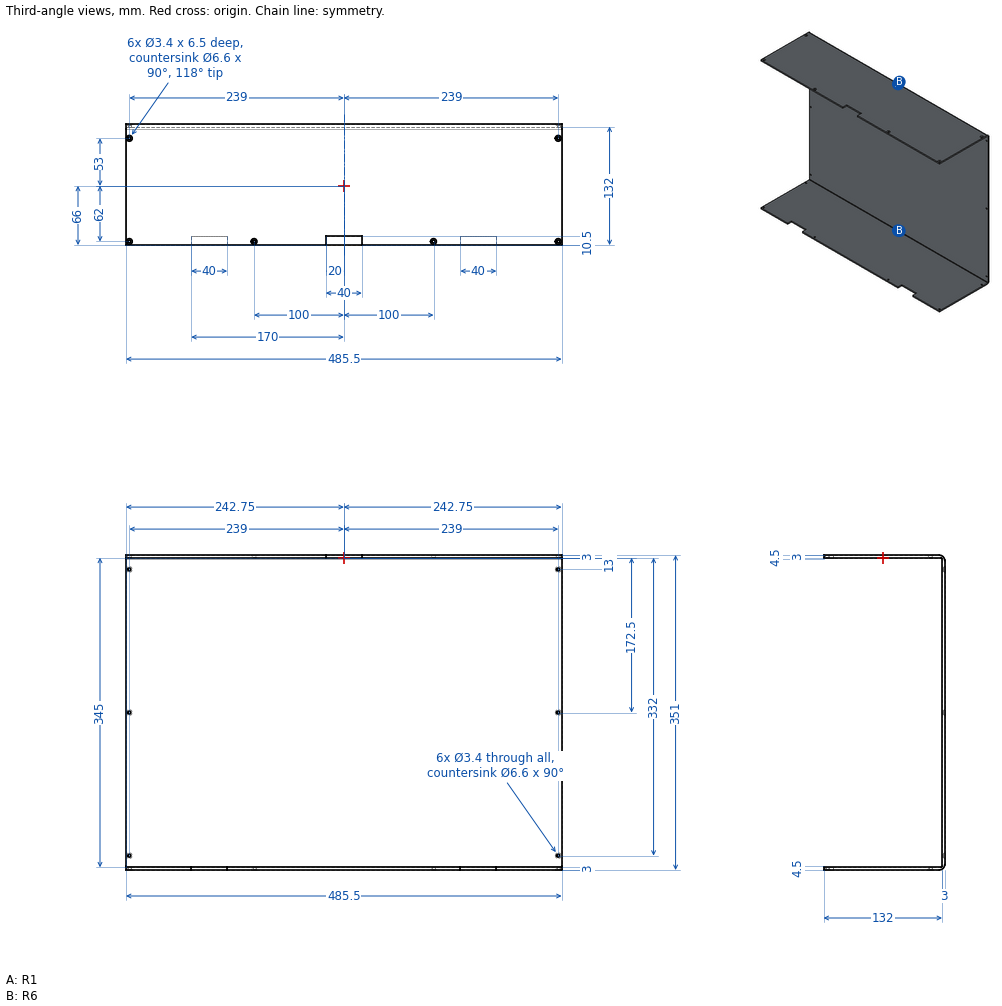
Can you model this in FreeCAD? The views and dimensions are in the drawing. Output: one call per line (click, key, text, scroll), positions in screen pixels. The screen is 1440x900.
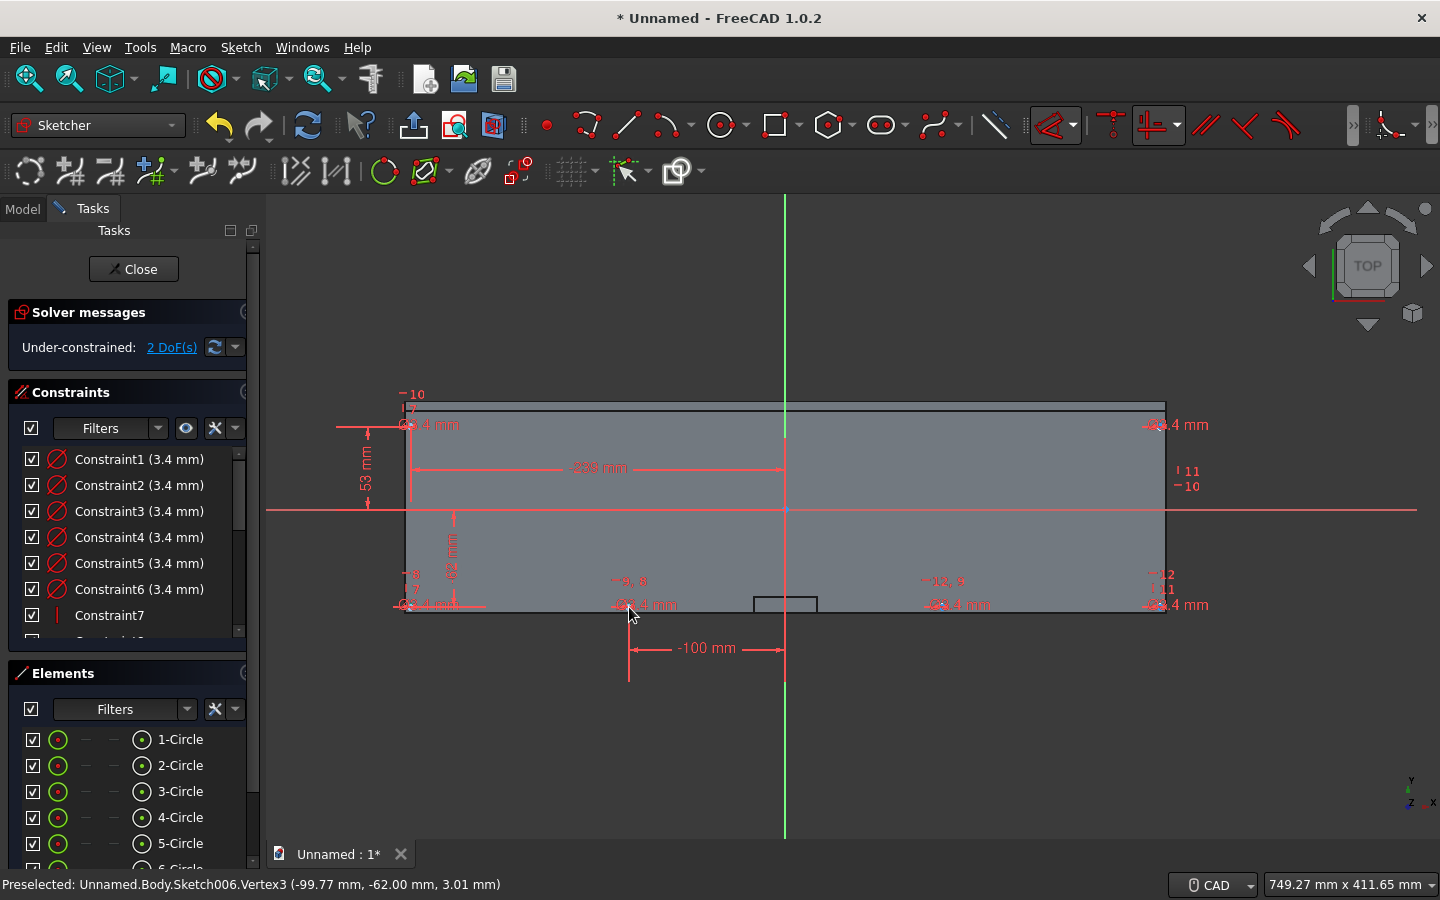
click(942, 607)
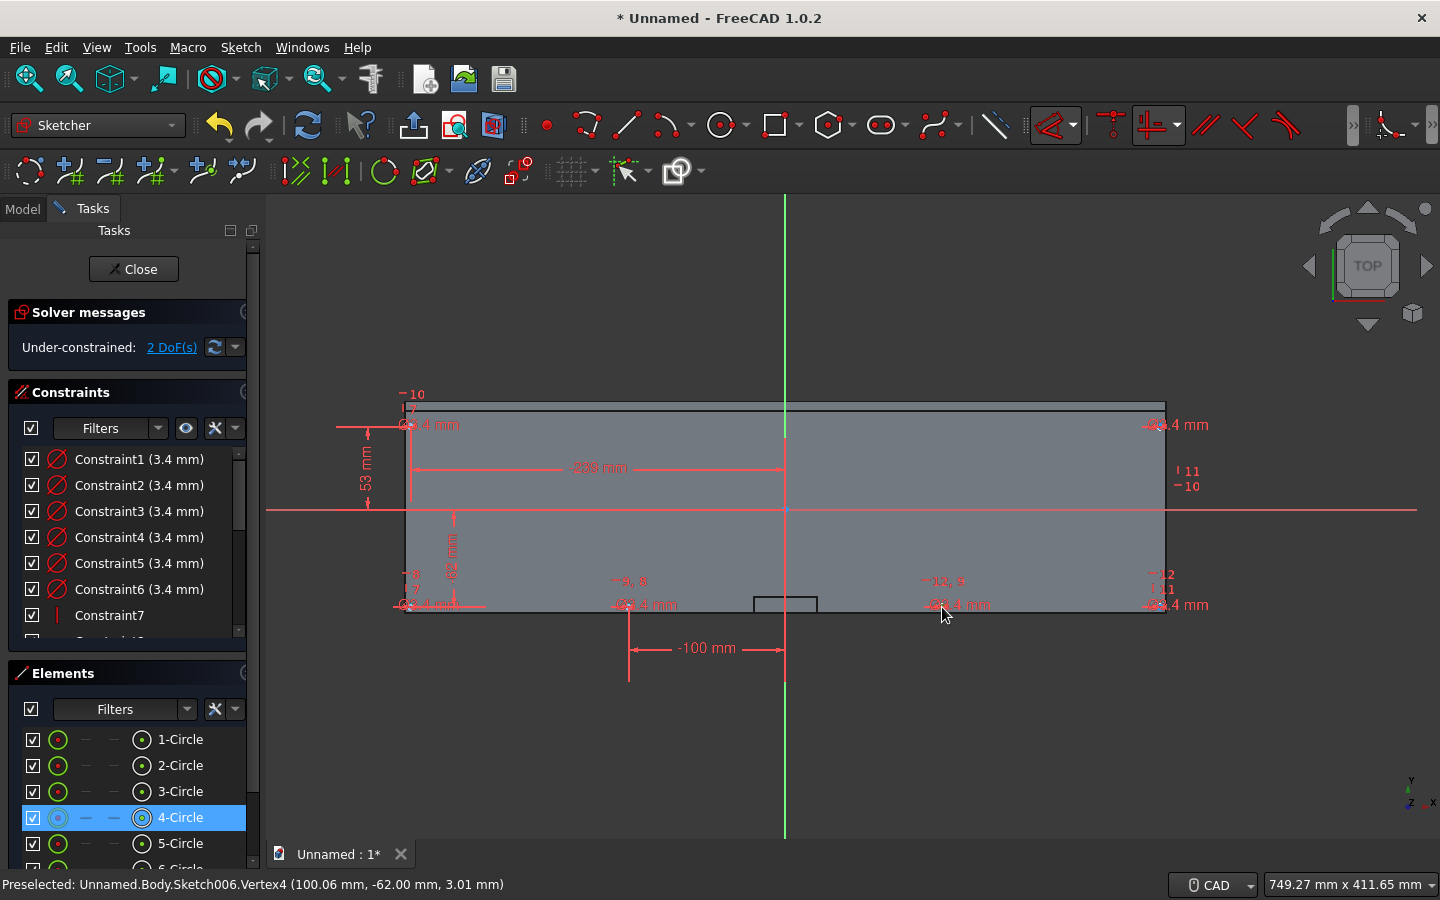
click(1076, 126)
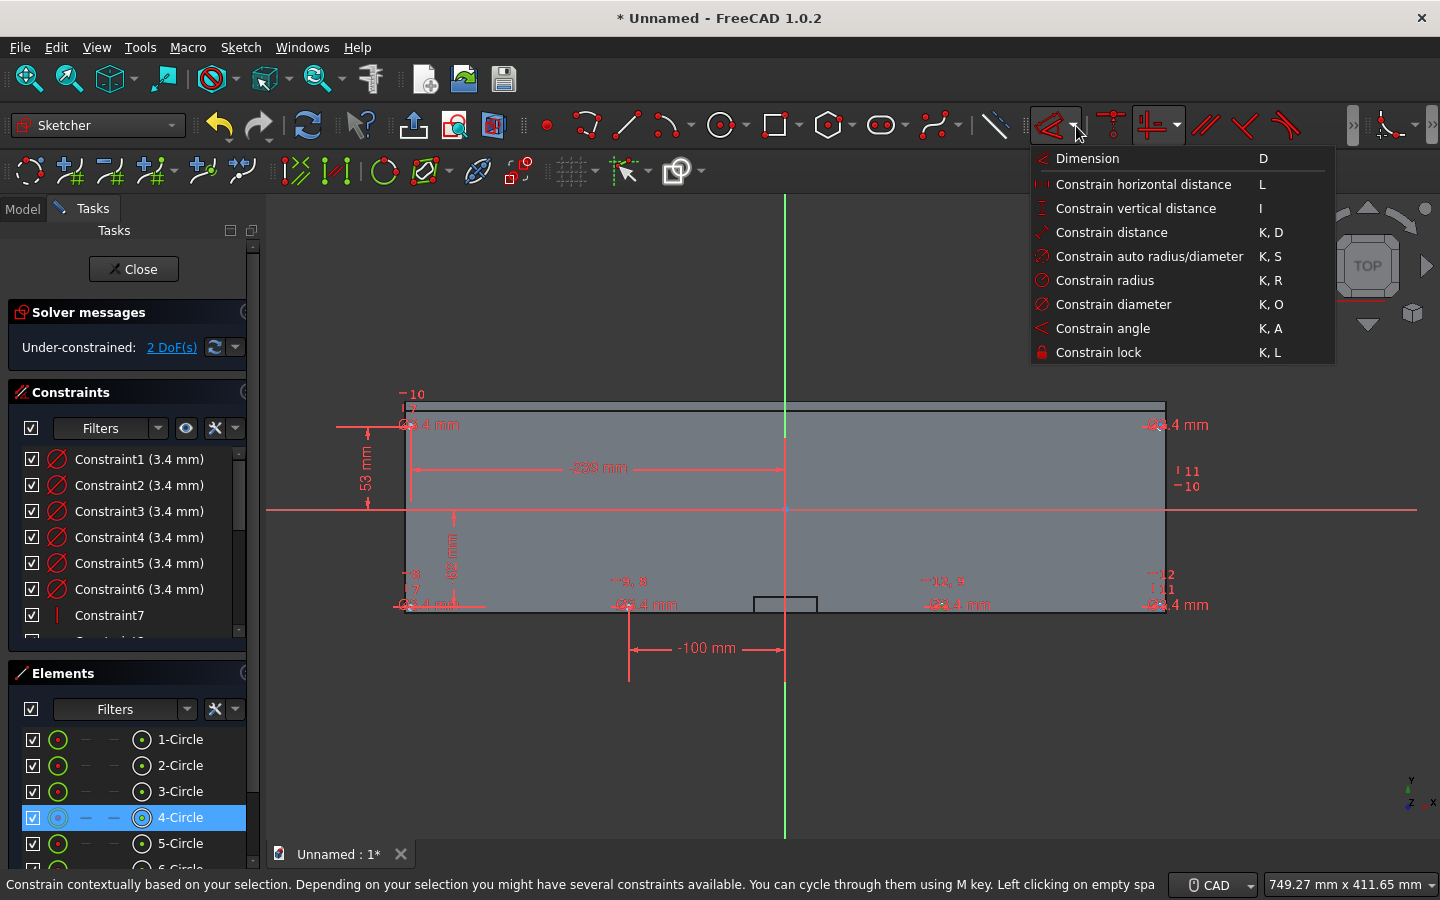
click(1183, 184)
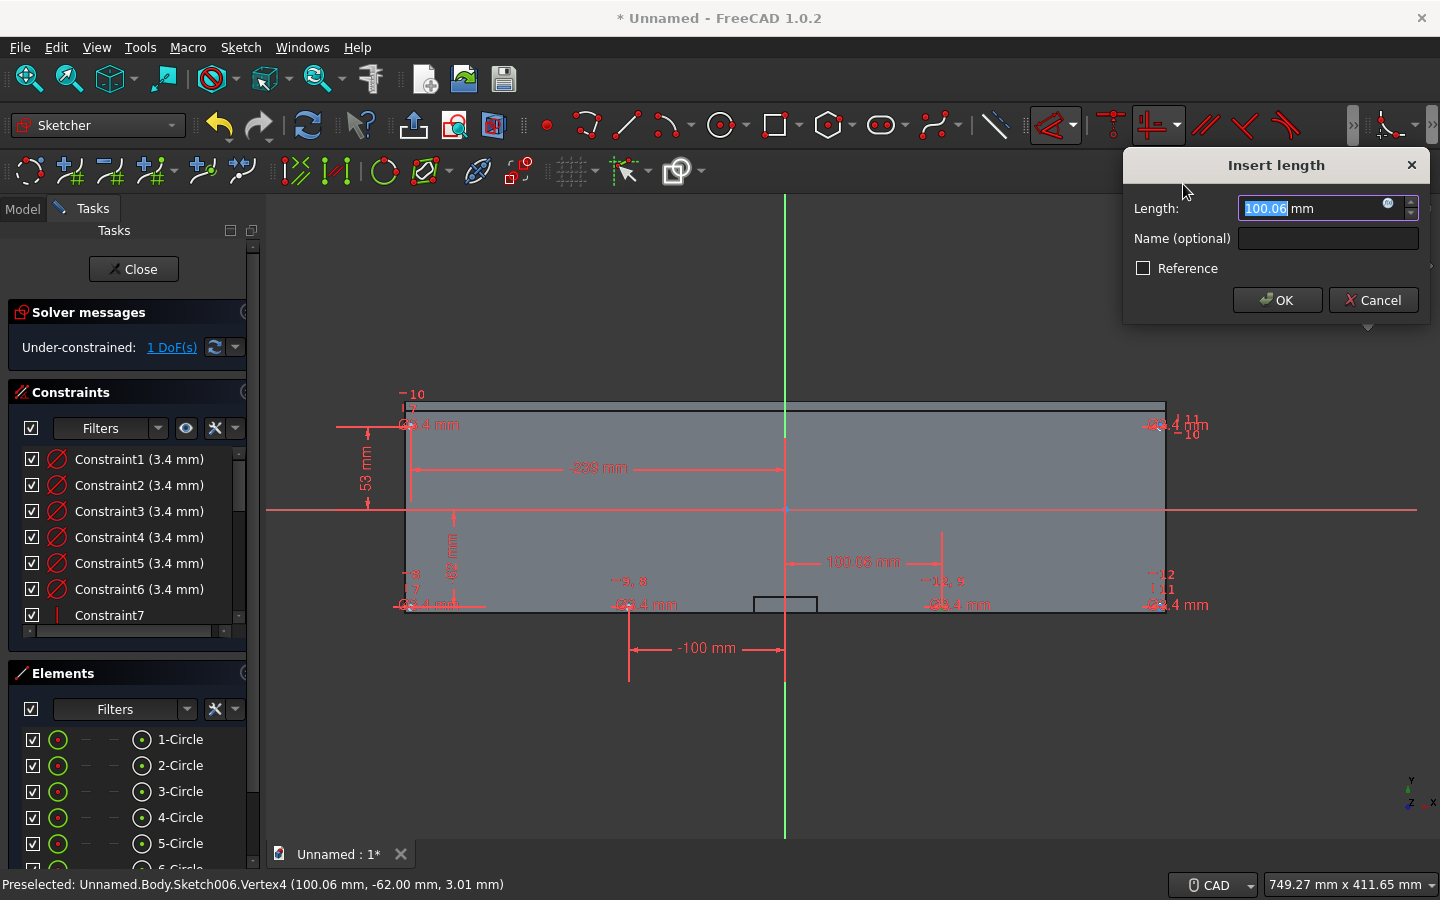
text(100)
key(Return)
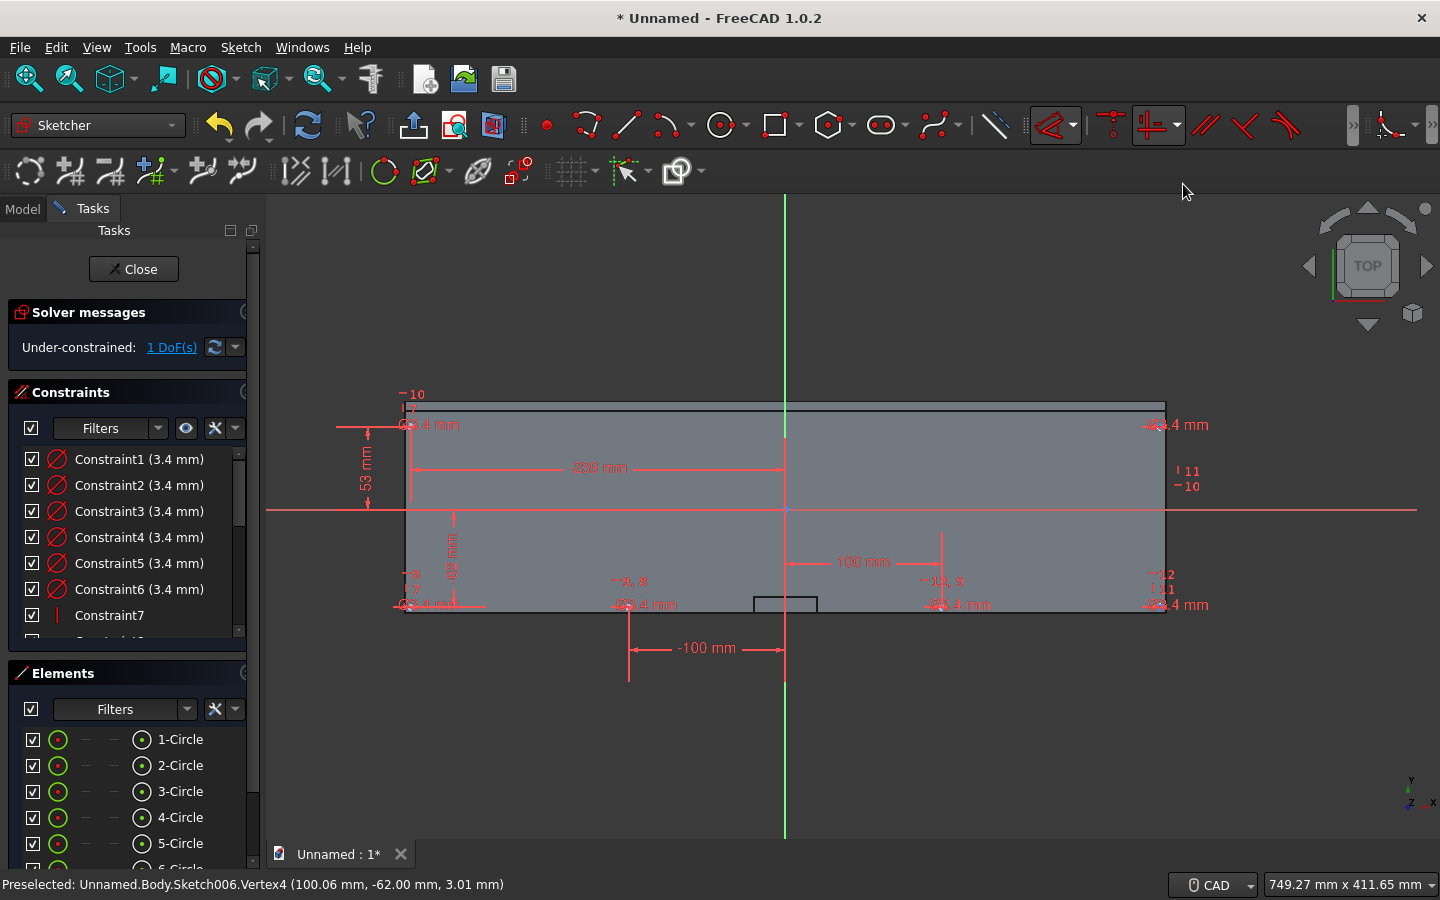
click(1160, 427)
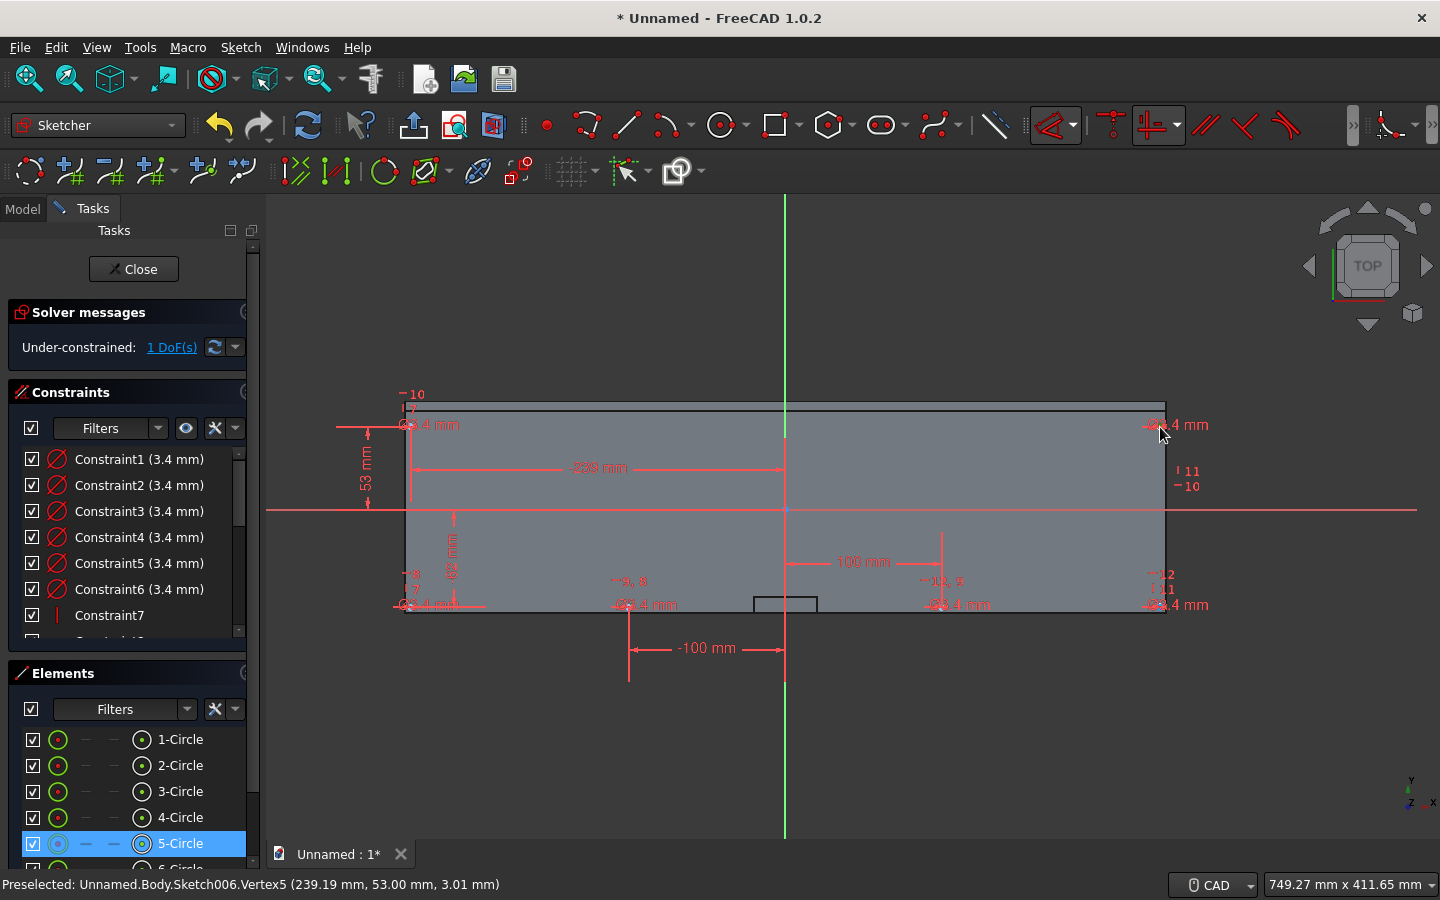
key(l)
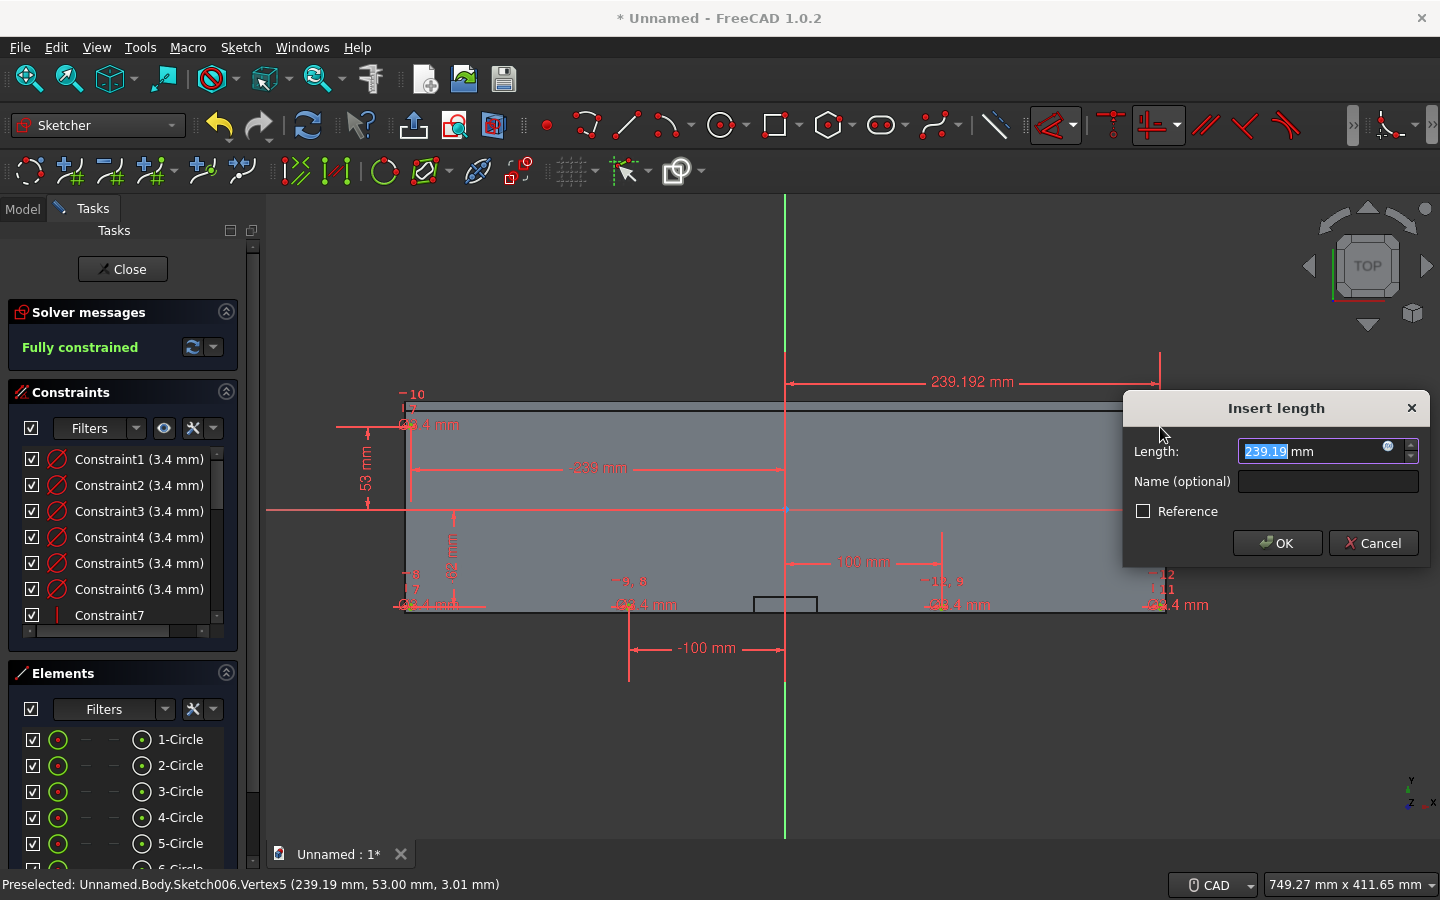
text(239)
key(Return)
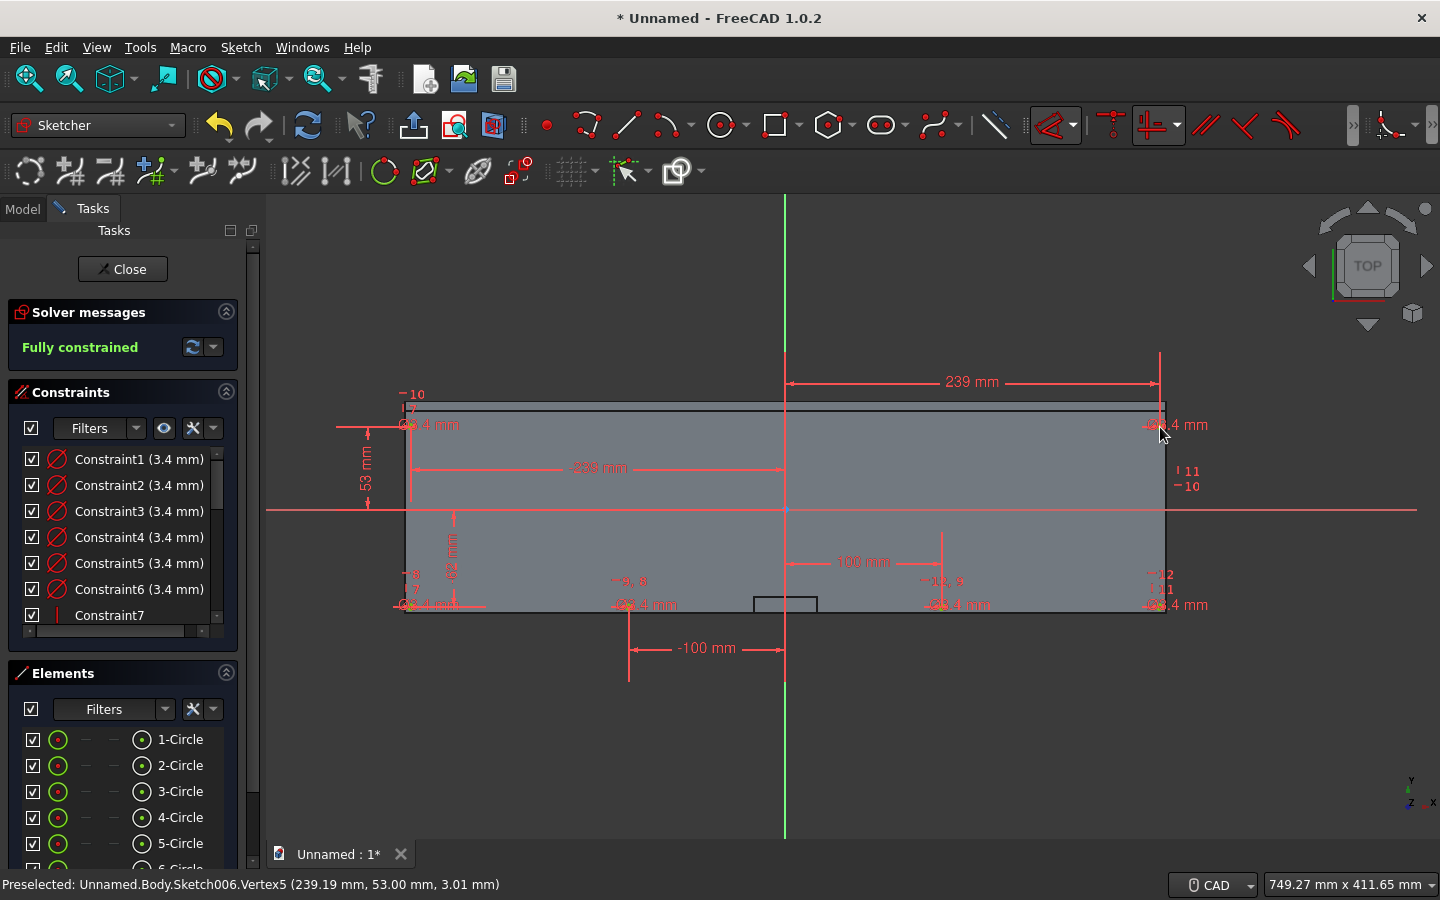
click(123, 269)